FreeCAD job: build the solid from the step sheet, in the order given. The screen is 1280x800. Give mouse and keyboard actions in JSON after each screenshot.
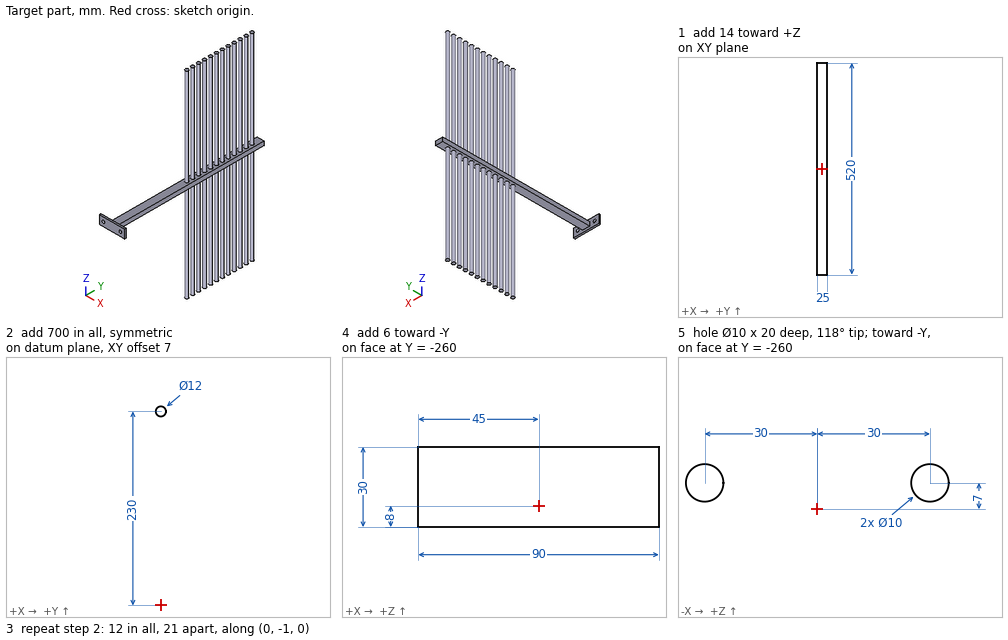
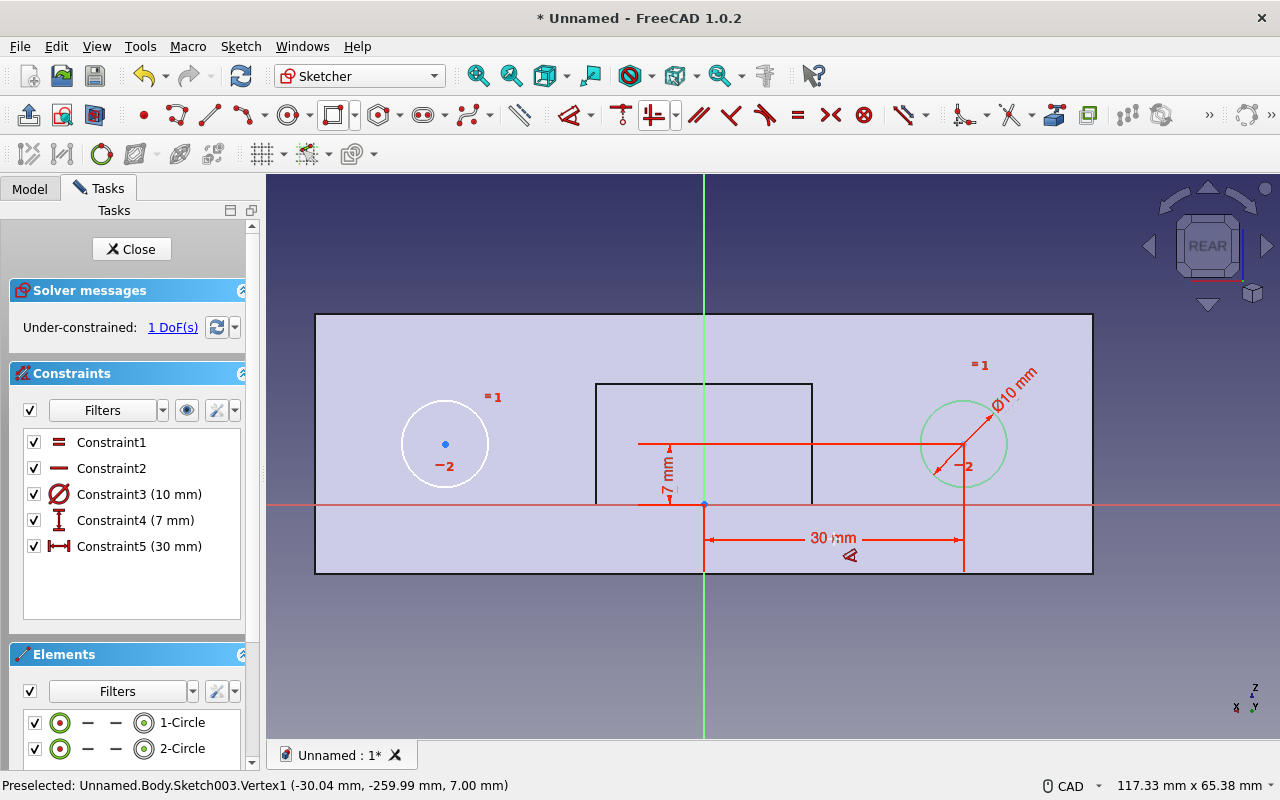
{"action": "left_click", "coordinate": [445, 444]}
{"action": "left_click", "coordinate": [575, 539]}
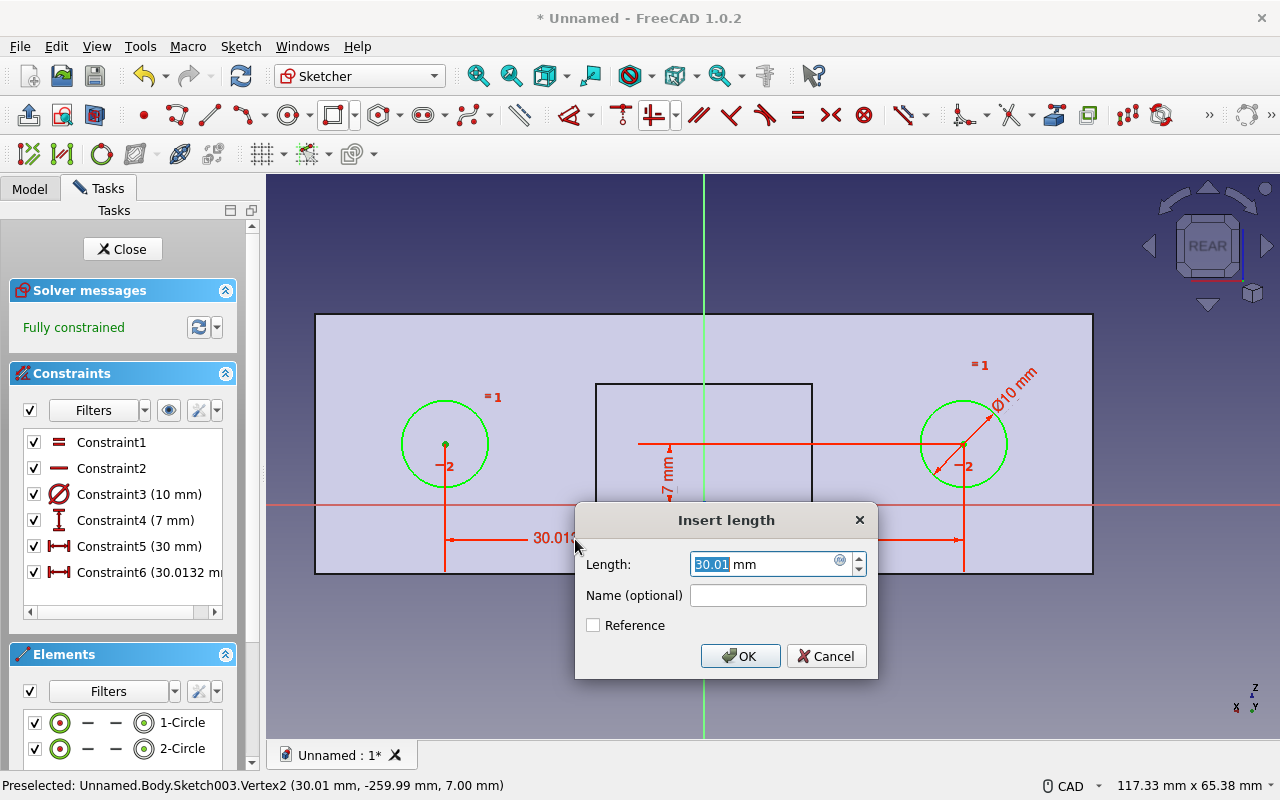
{"action": "type", "text": "30"}
{"action": "key", "text": "Return"}
{"action": "key", "text": "Escape"}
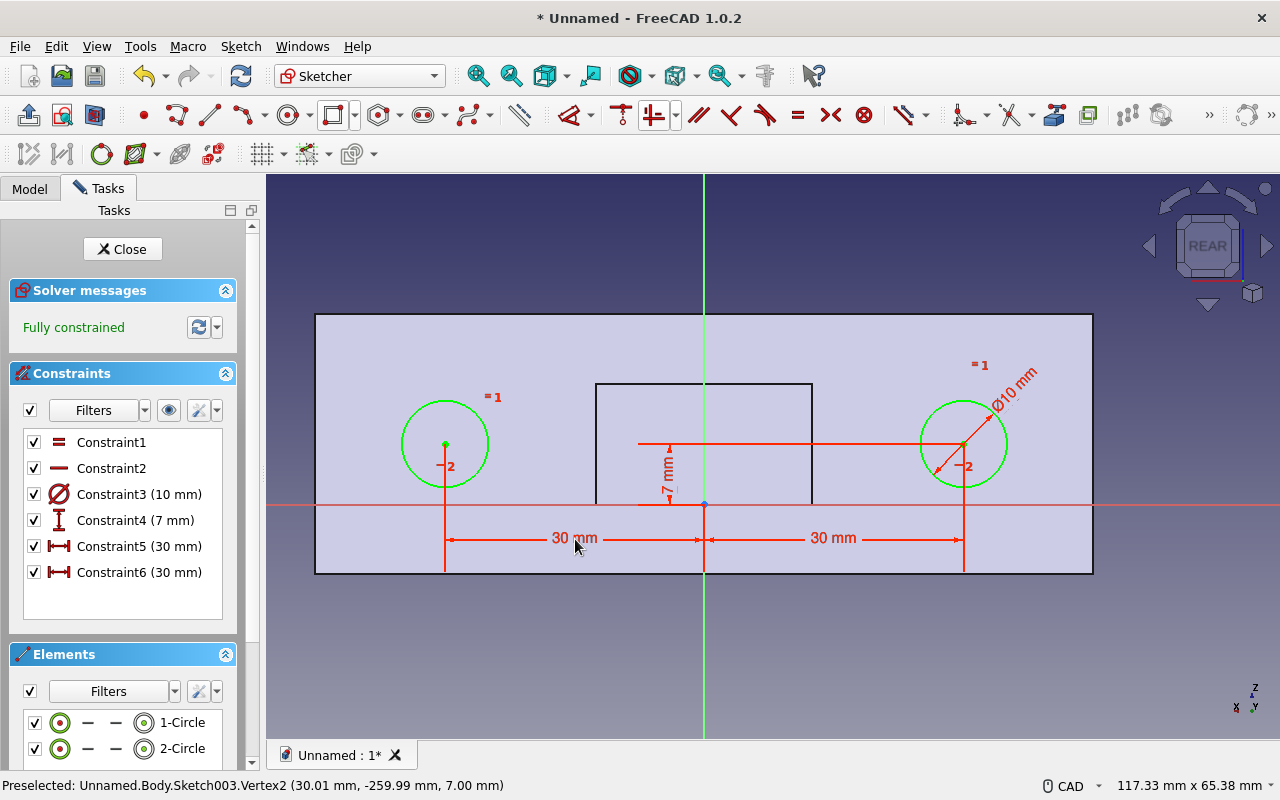
{"action": "left_click", "coordinate": [123, 249]}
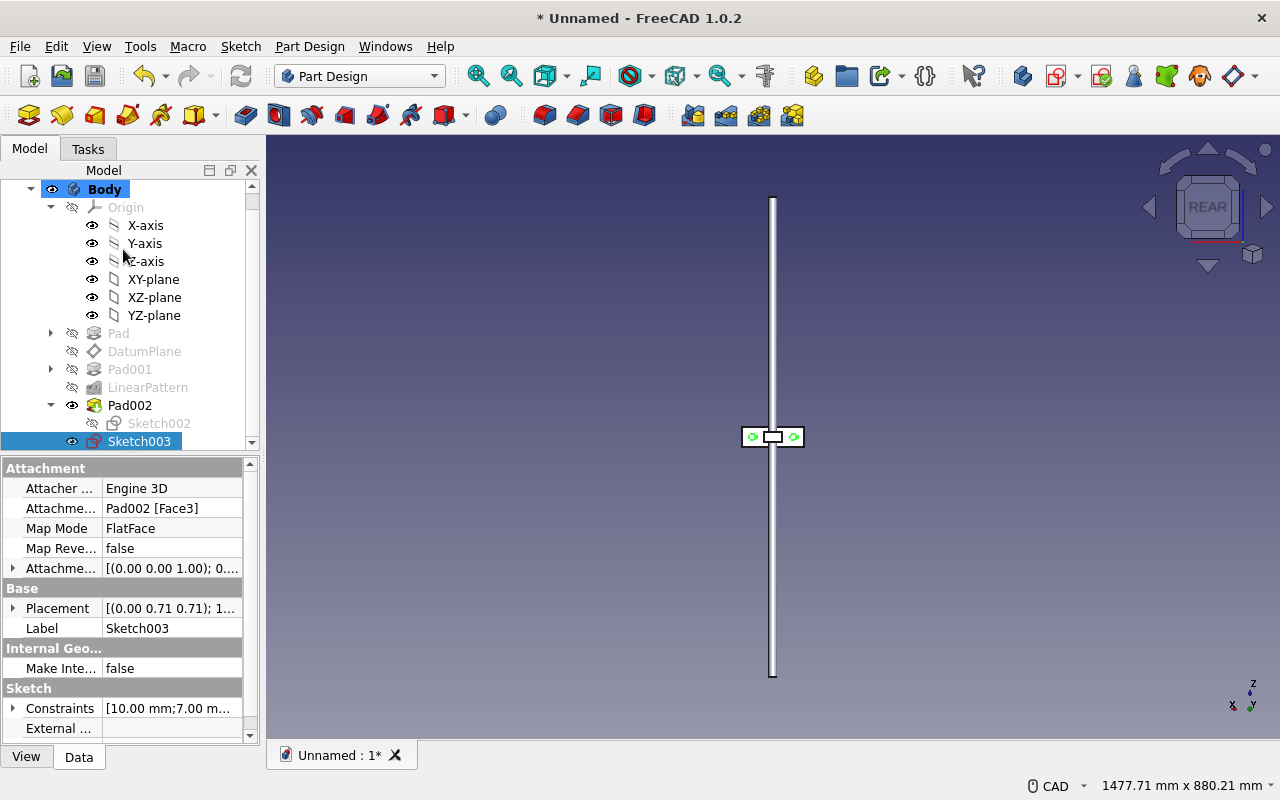
{"action": "left_click", "coordinate": [279, 116]}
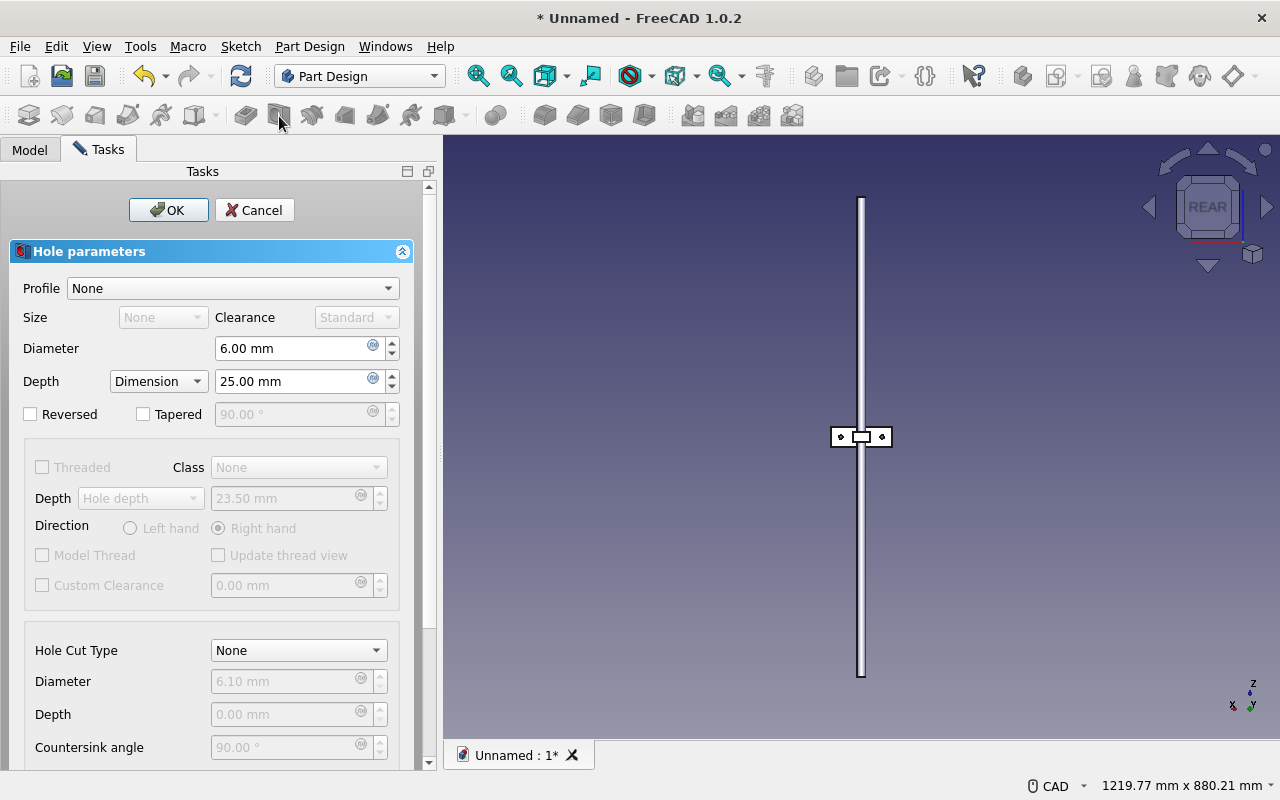
{"action": "triple_click", "coordinate": [300, 348]}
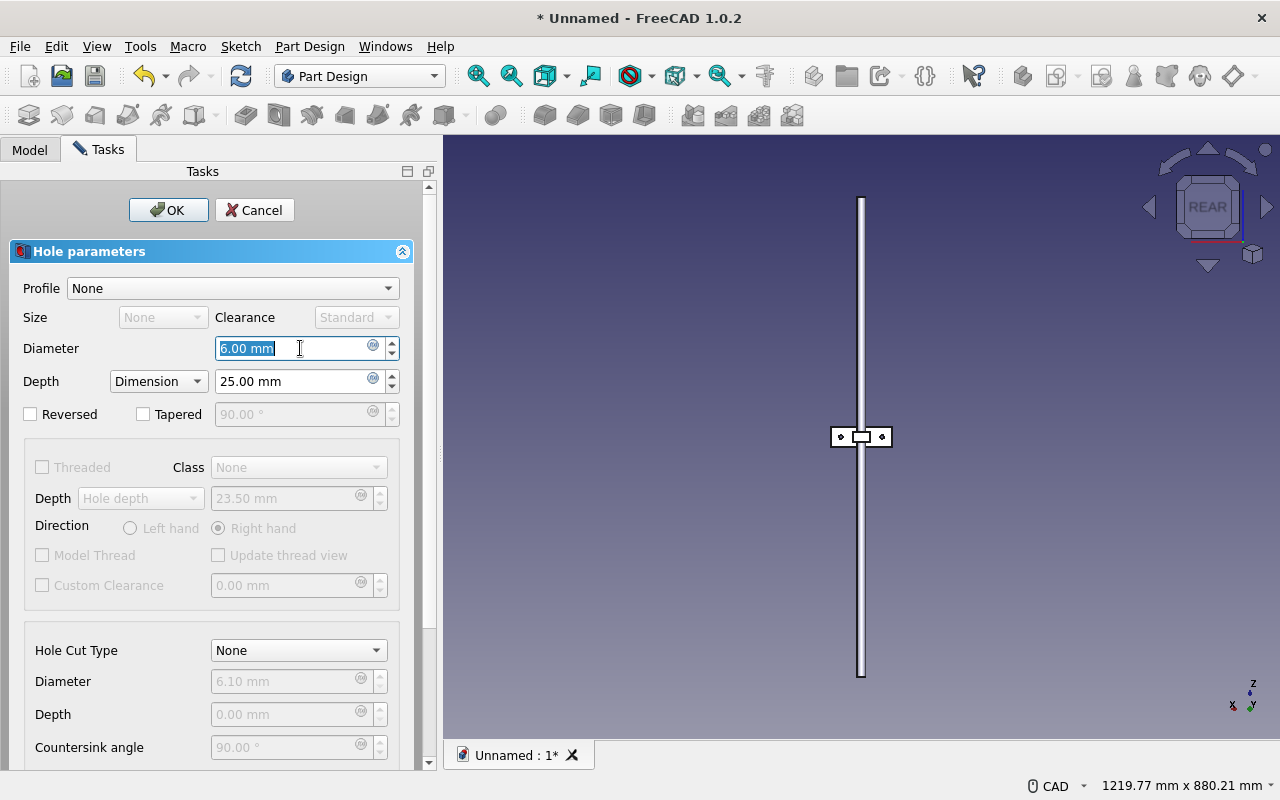
{"action": "type", "text": "10"}
{"action": "key", "text": "Tab"}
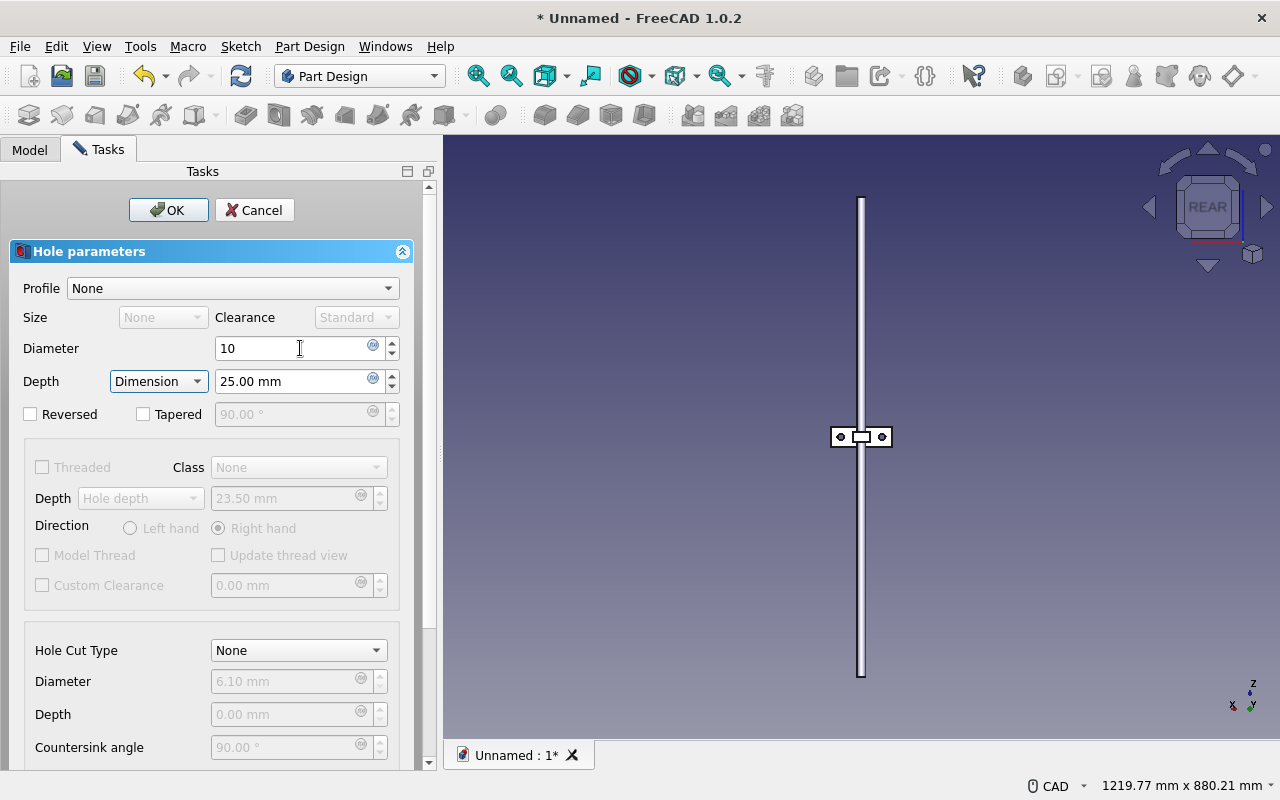
{"action": "triple_click", "coordinate": [300, 382]}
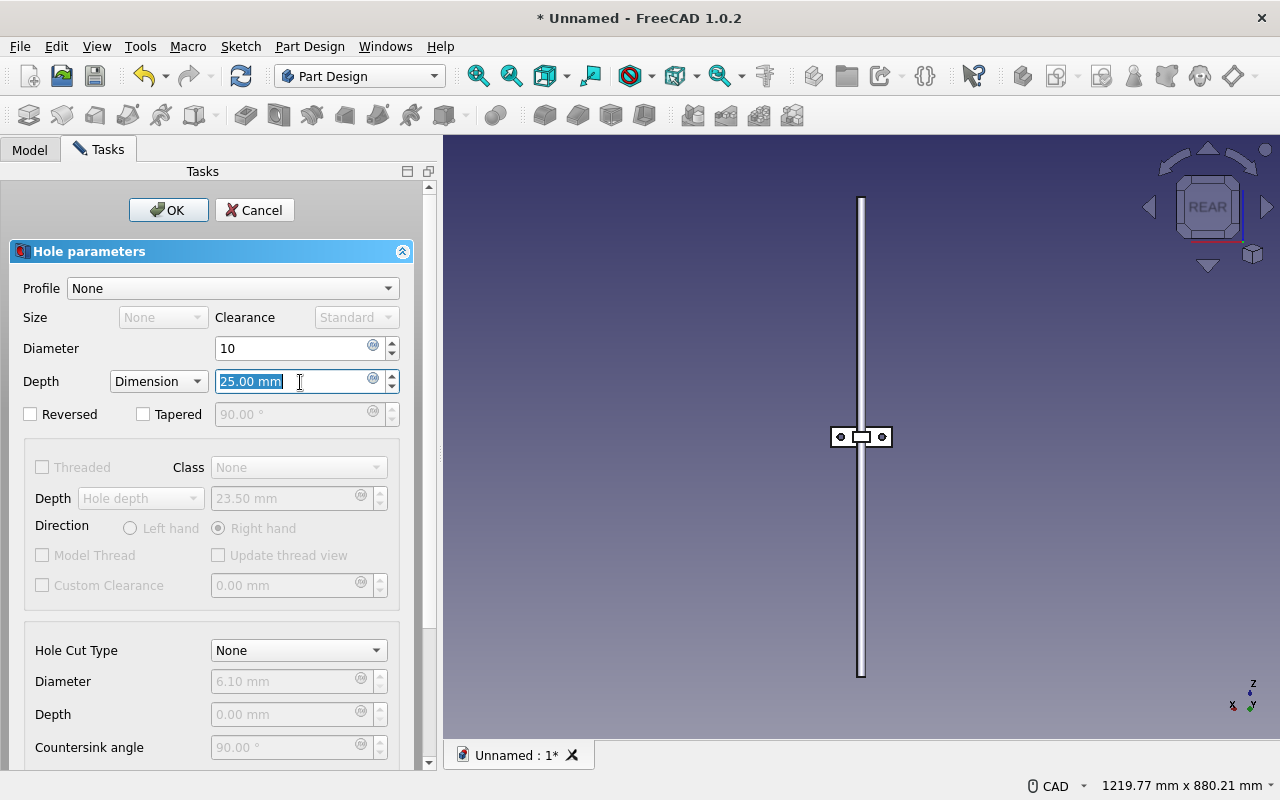
{"action": "type", "text": "20"}
{"action": "key", "text": "Tab"}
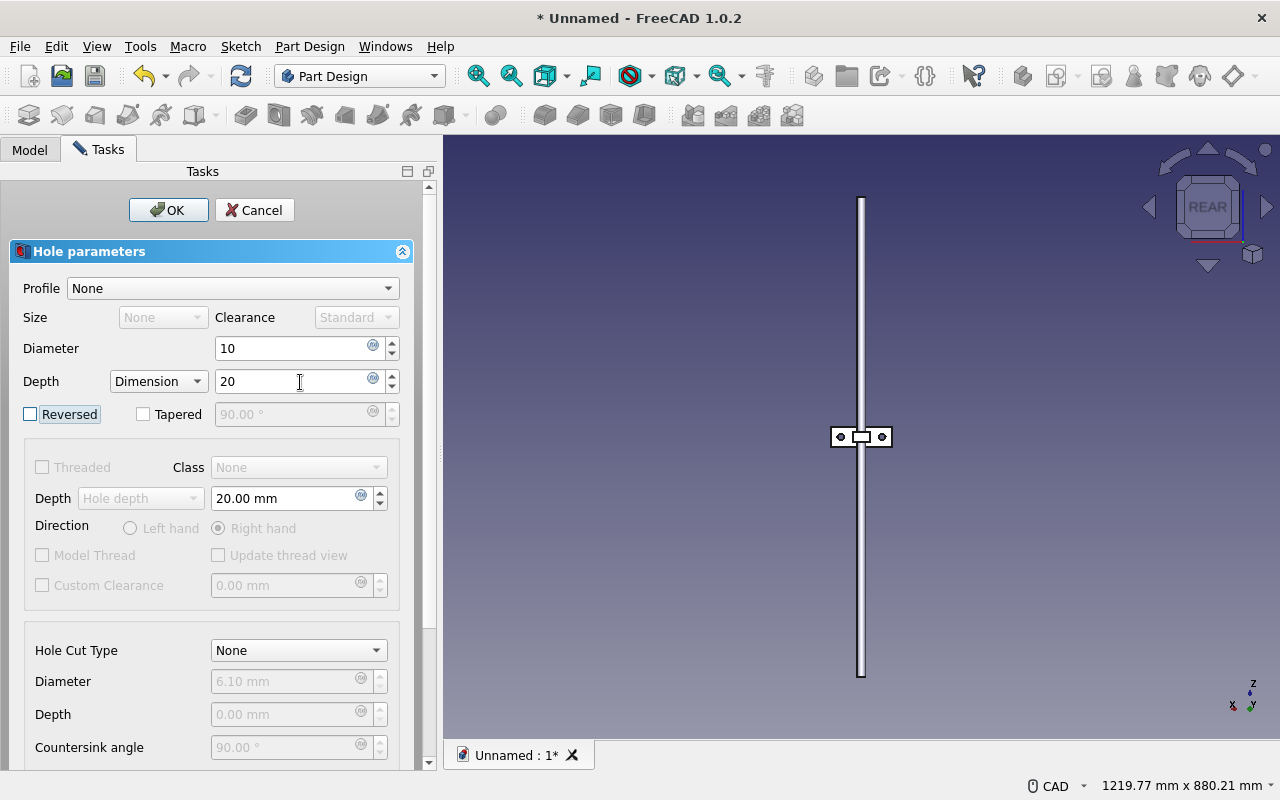
{"action": "left_click", "coordinate": [169, 210]}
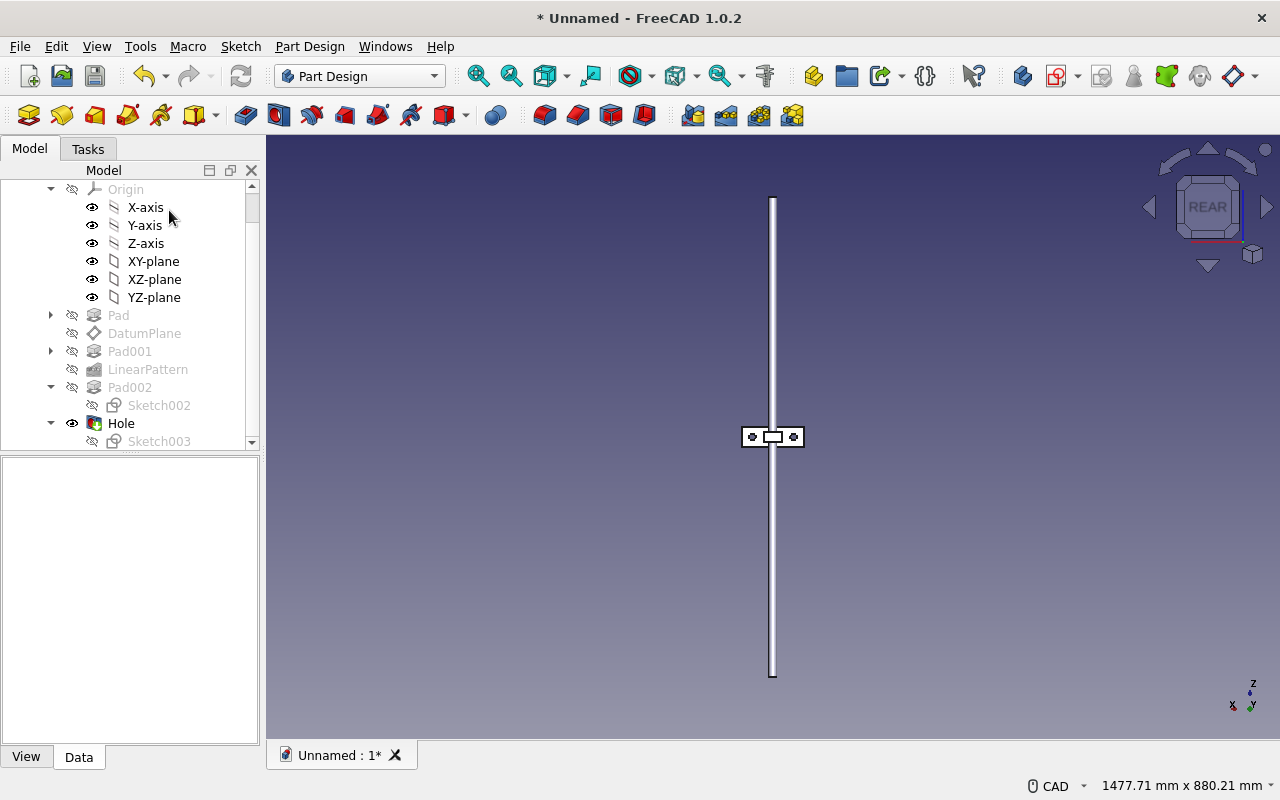
{"action": "key", "text": "0"}